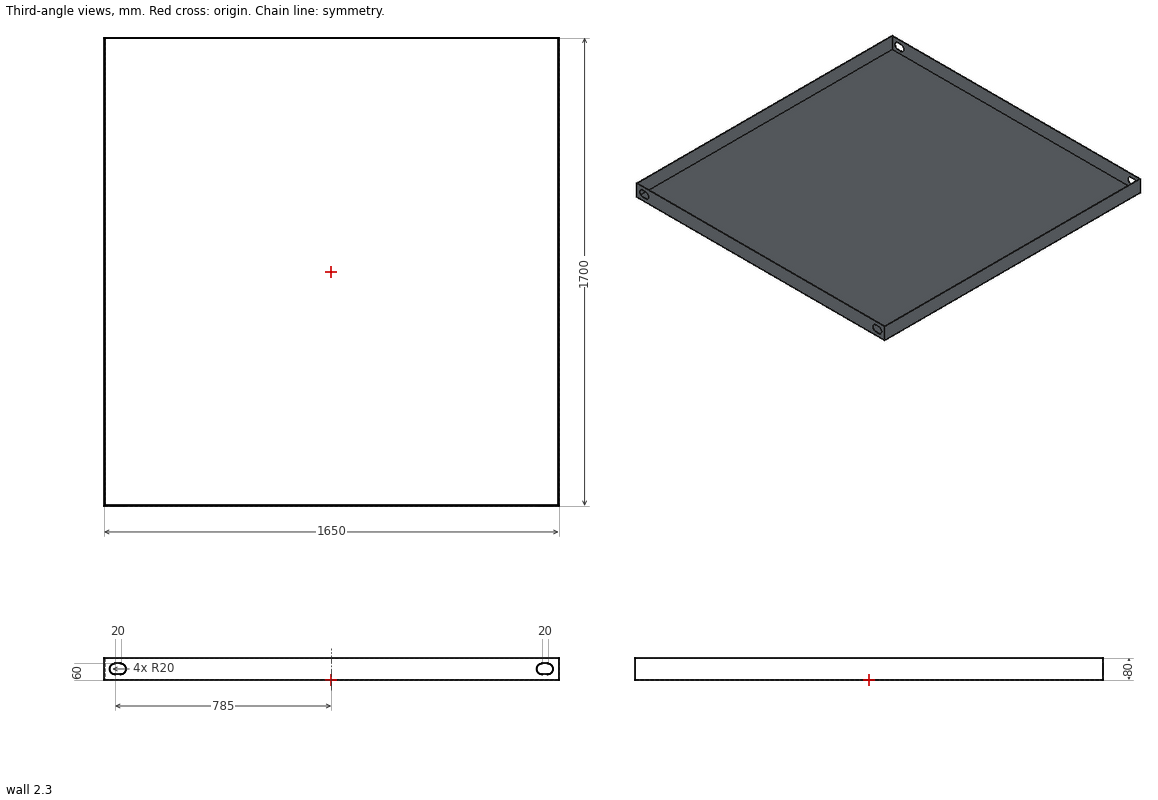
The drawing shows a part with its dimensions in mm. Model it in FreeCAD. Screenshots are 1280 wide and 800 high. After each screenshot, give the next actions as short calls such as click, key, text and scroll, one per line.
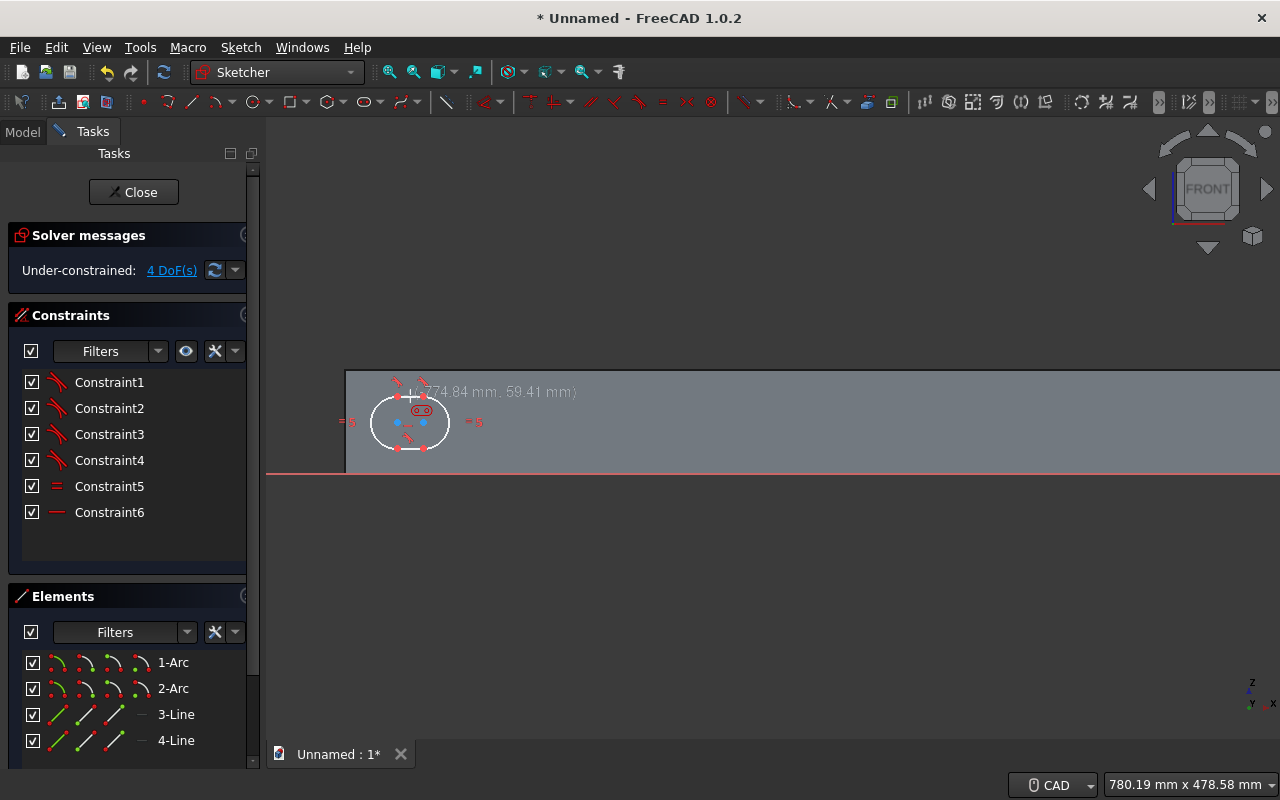
scroll(397, 425, down, 6)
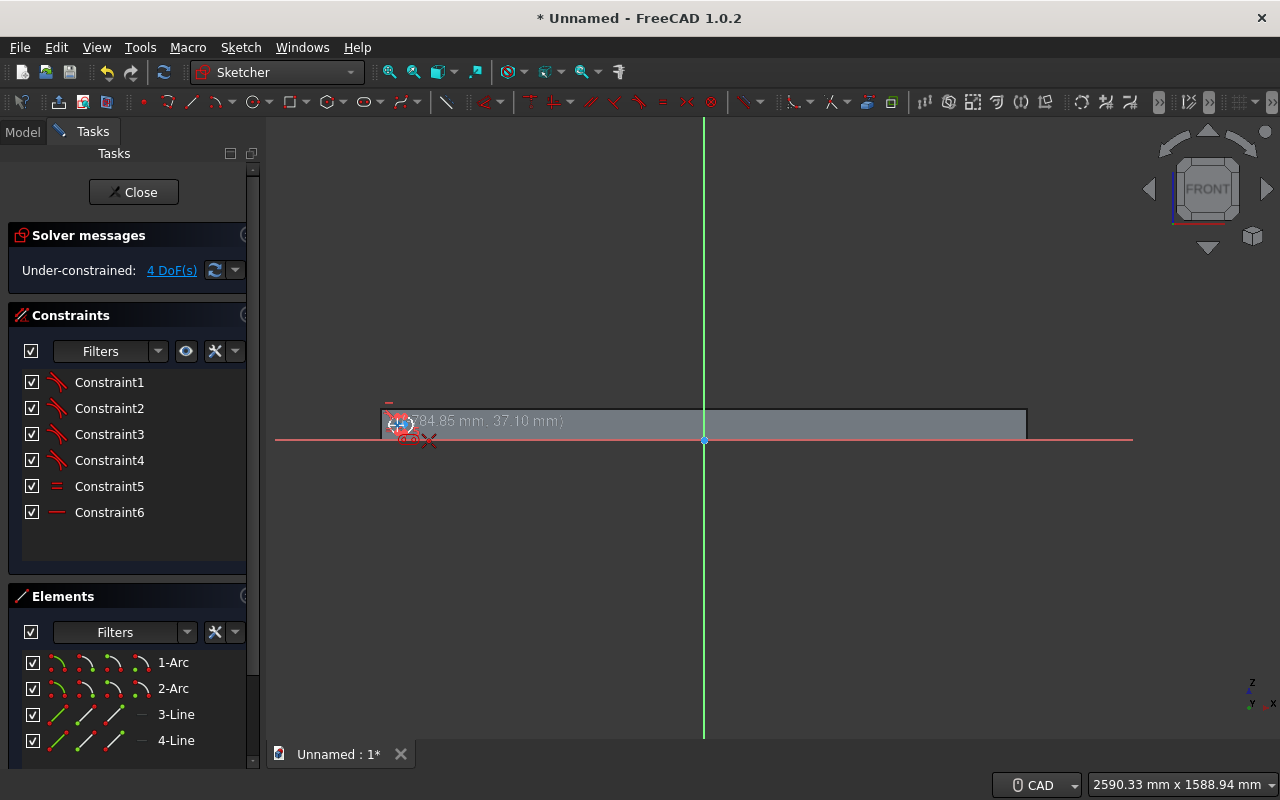
scroll(1004, 425, up, 6)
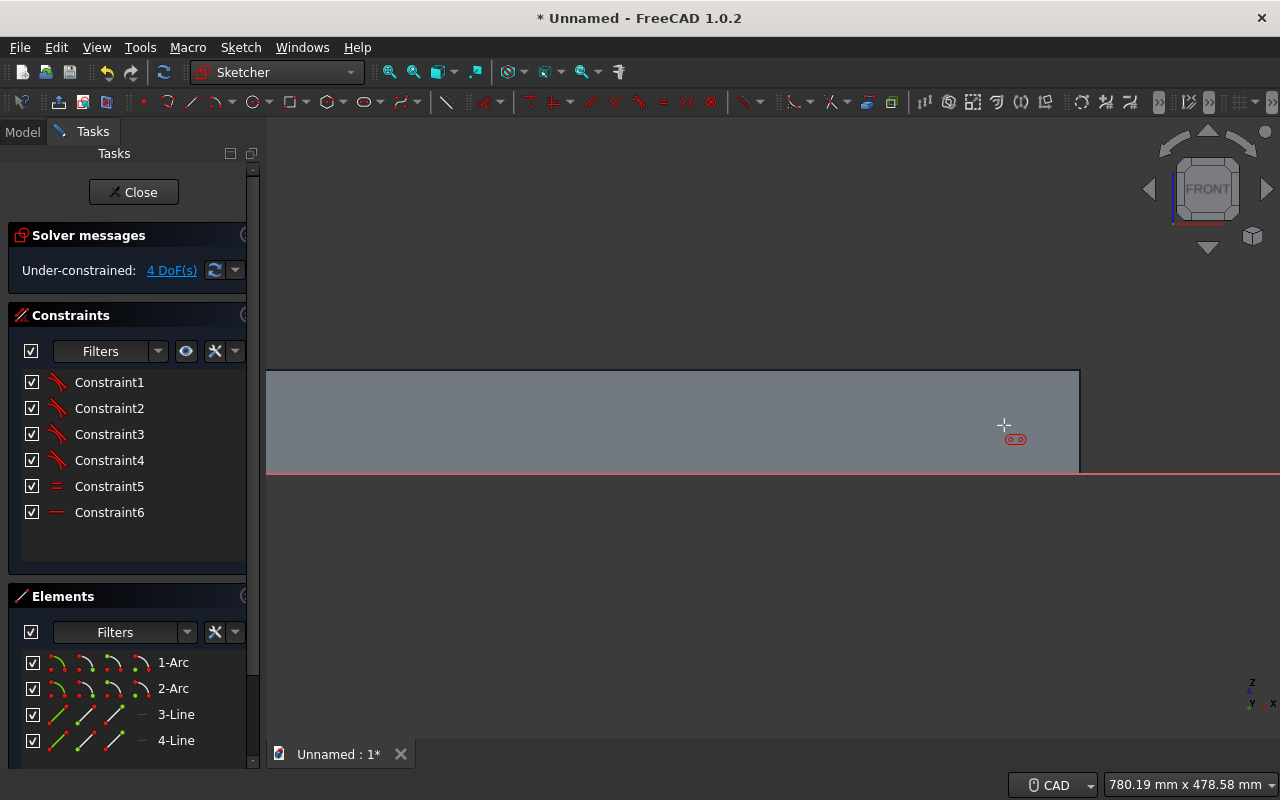
click(1002, 422)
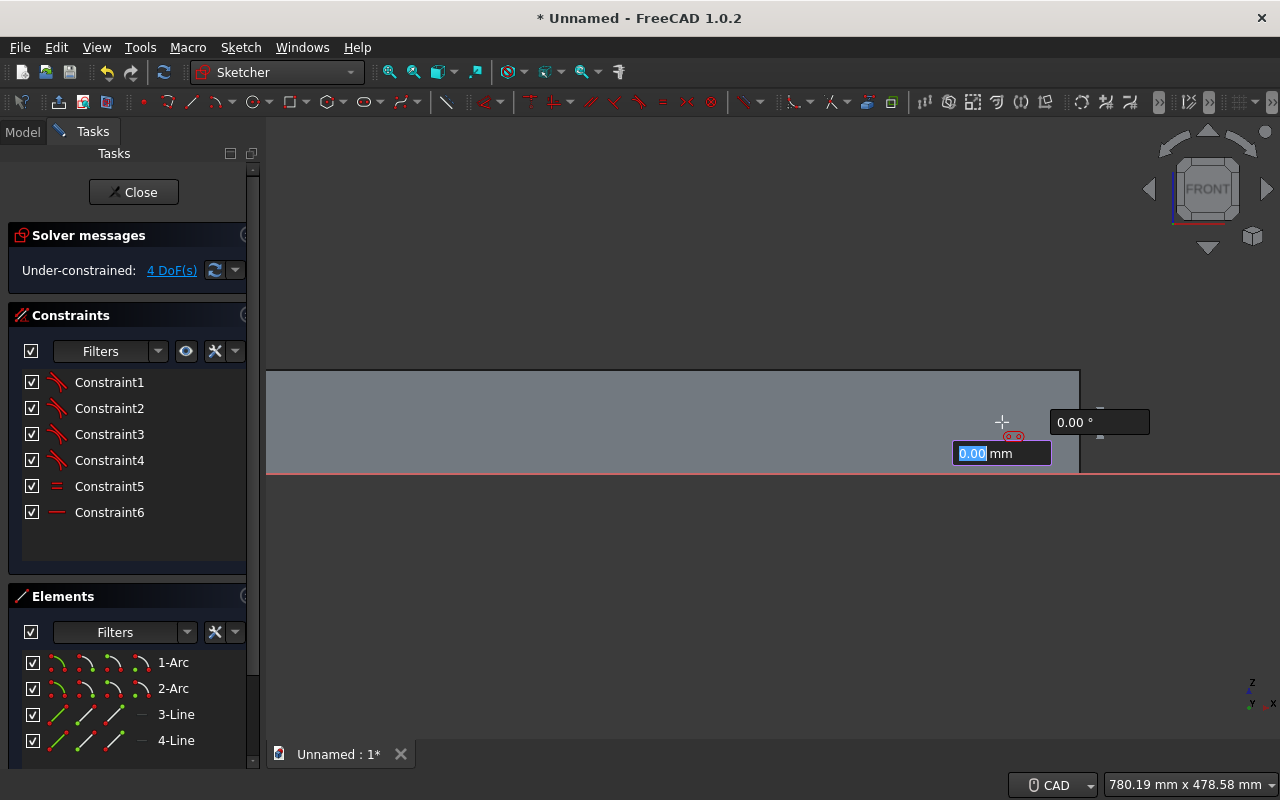
click(1028, 422)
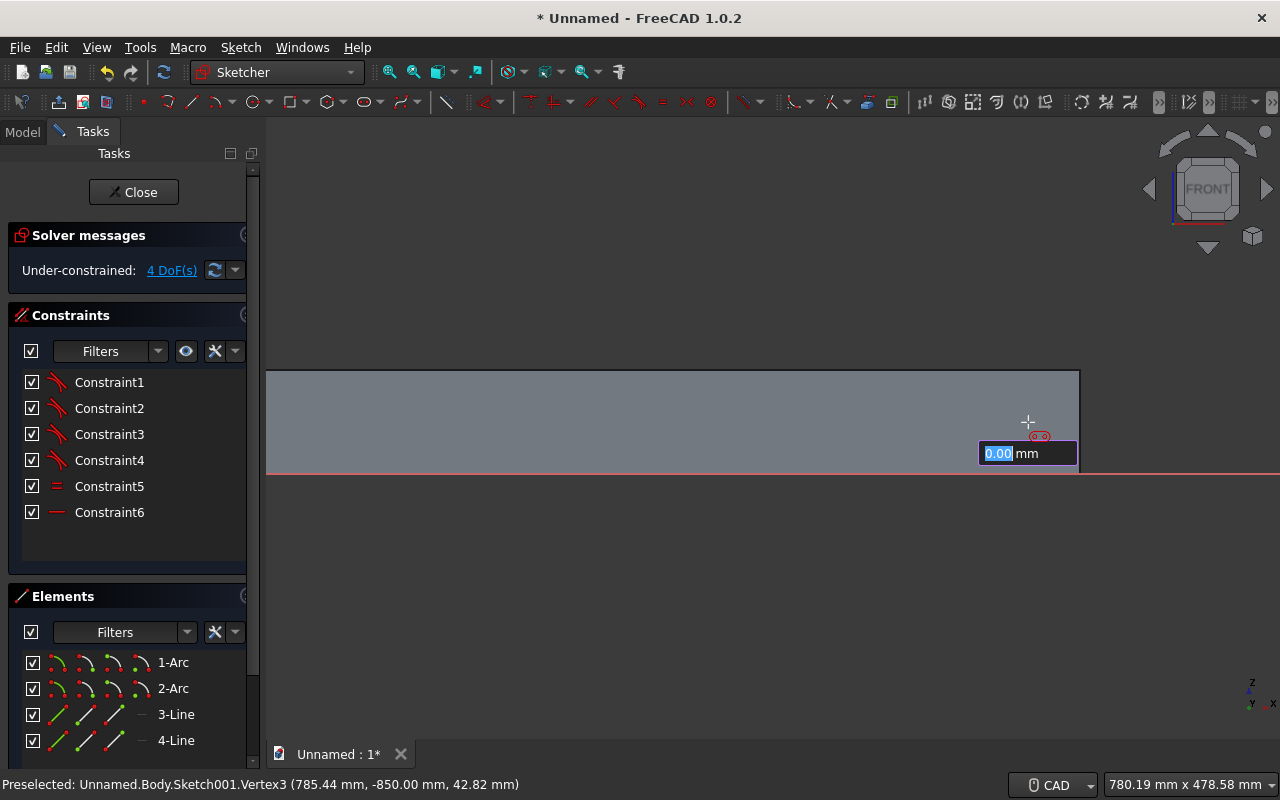
click(1015, 396)
key(Escape)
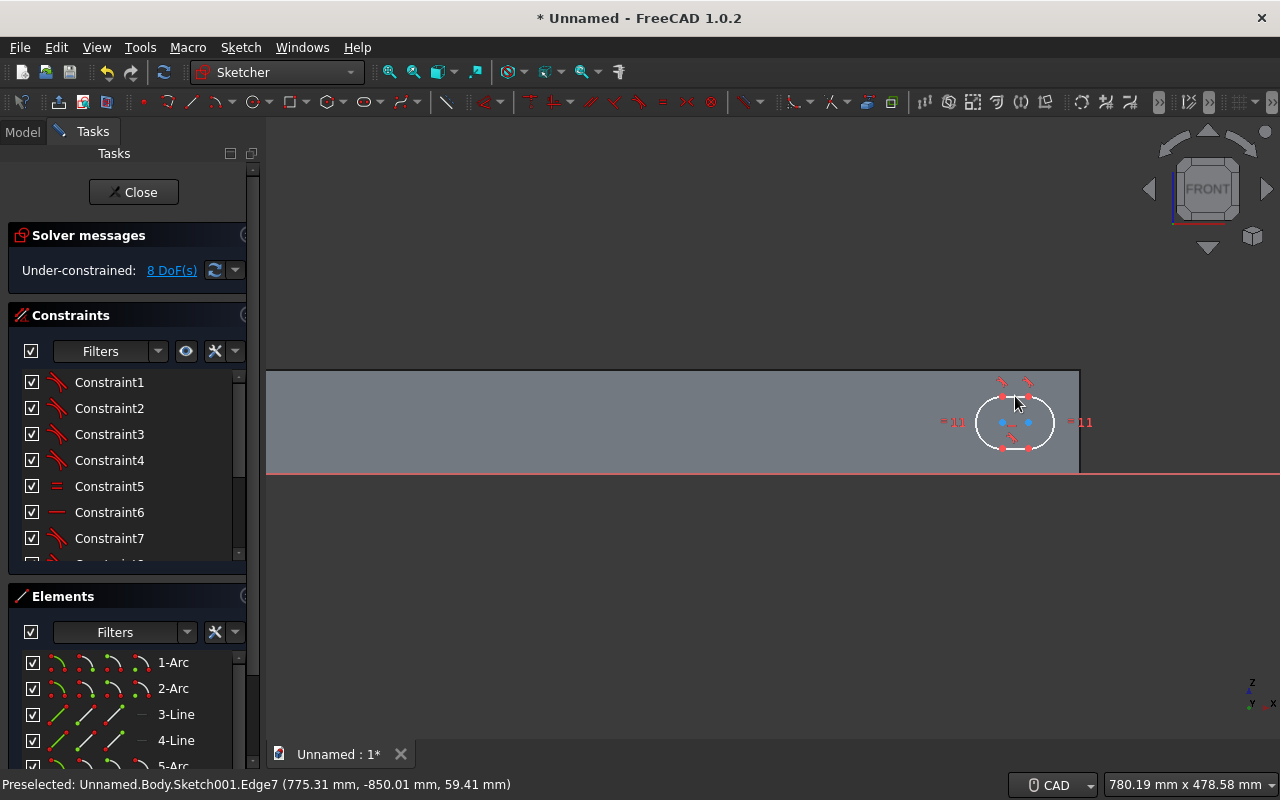
scroll(1005, 425, down, 6)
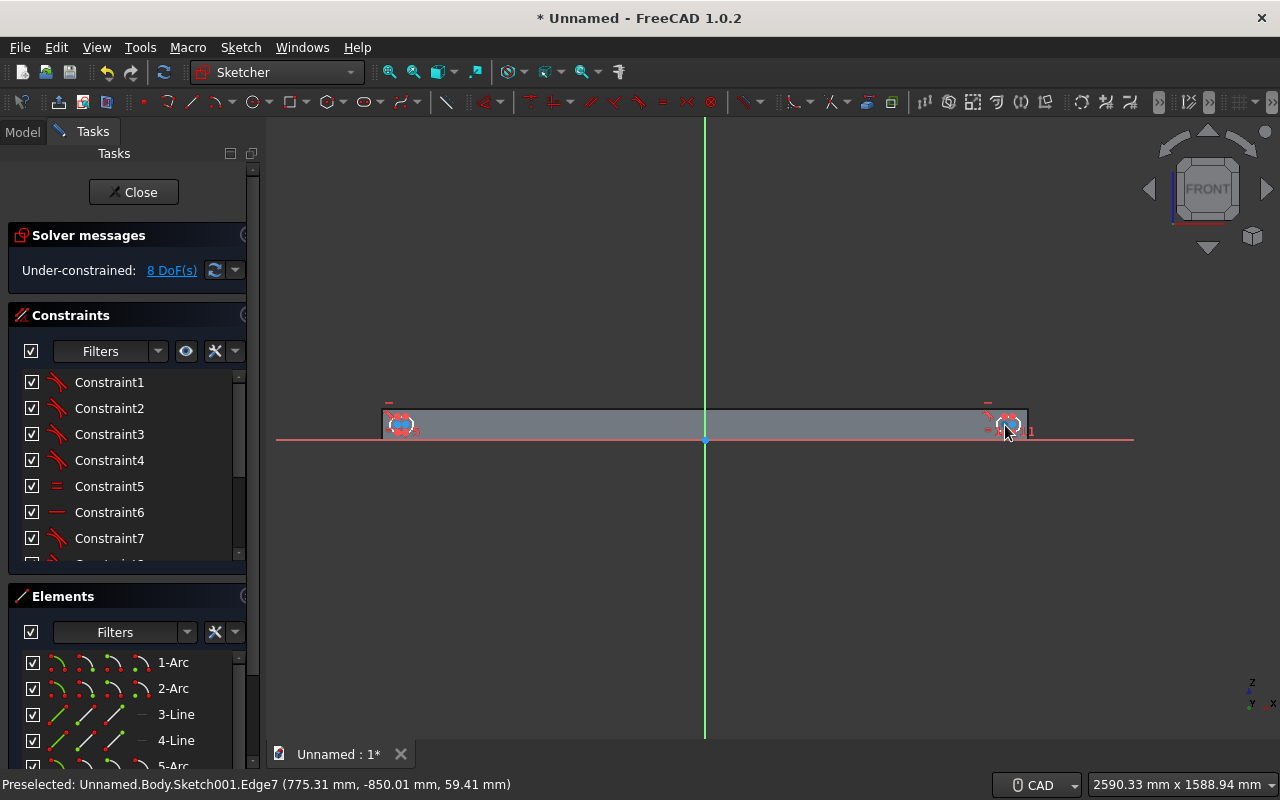
scroll(391, 420, up, 4)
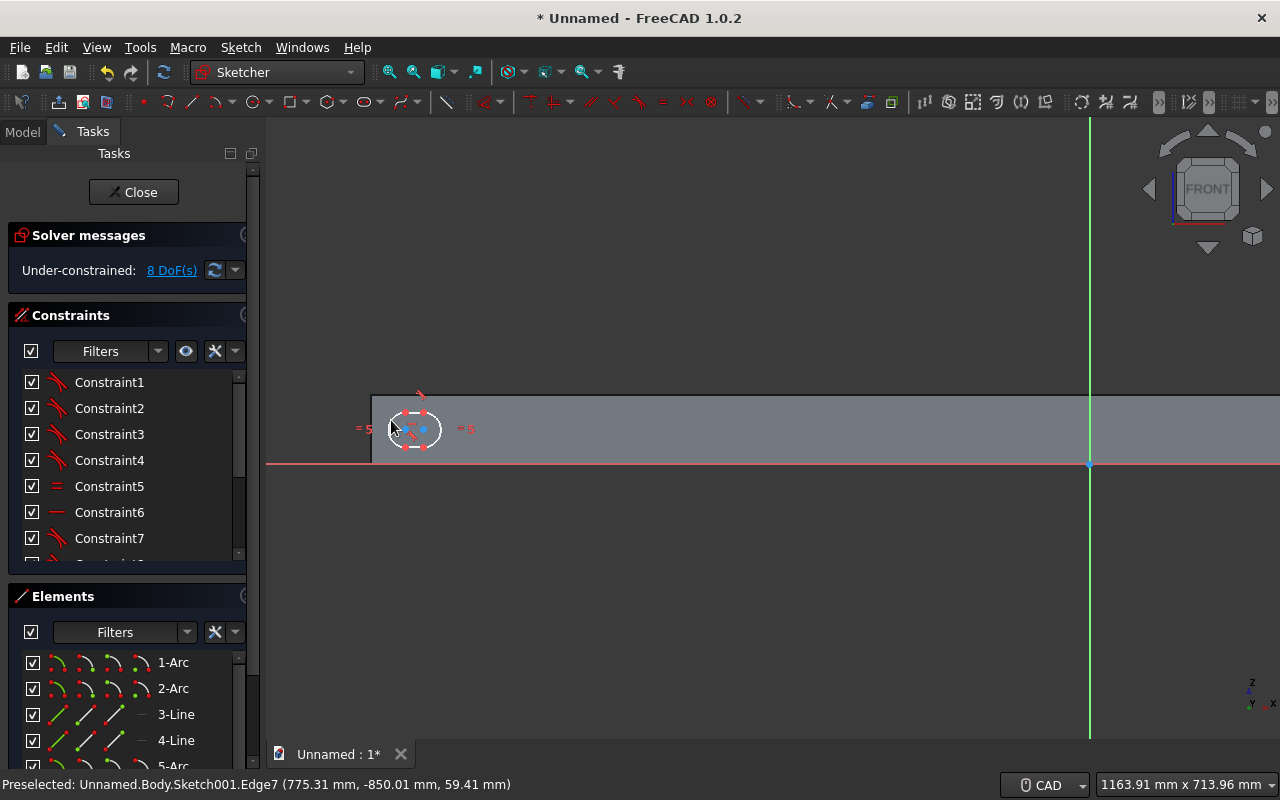
click(392, 420)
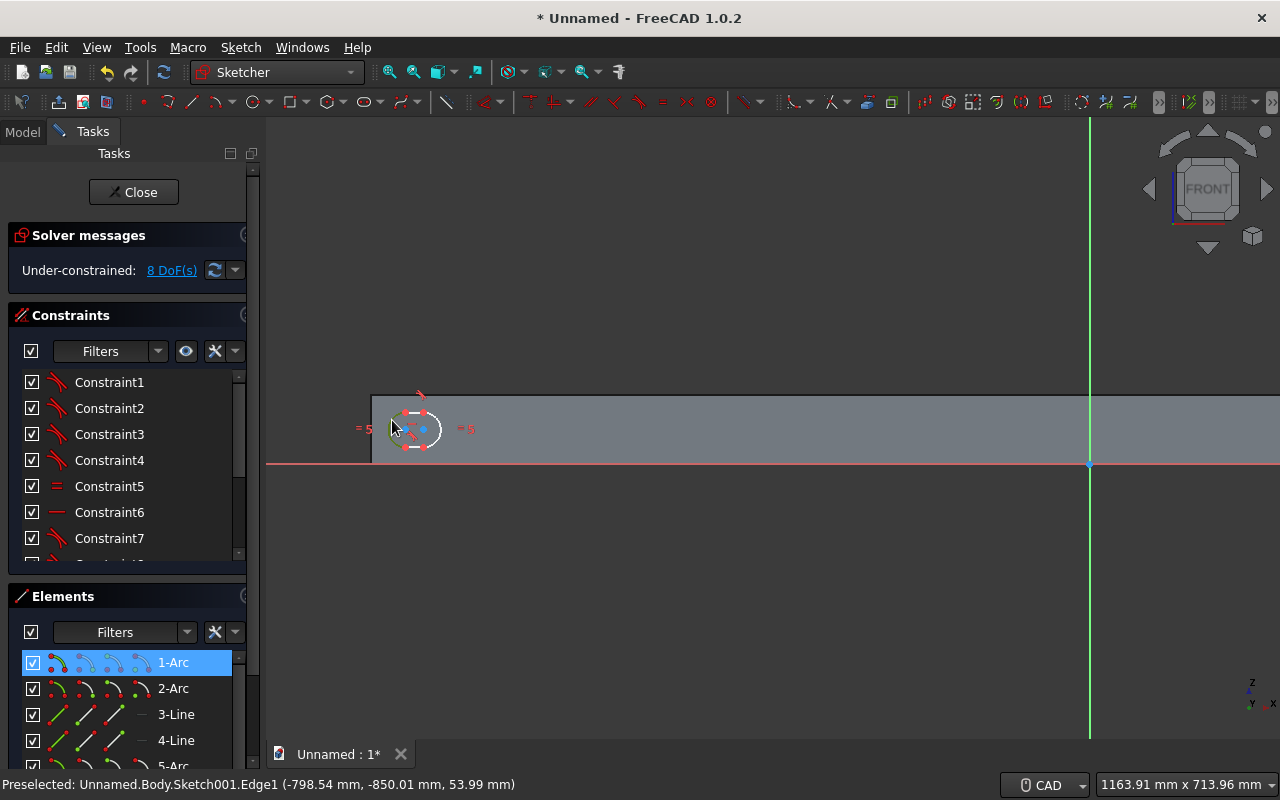
scroll(390, 420, down, 4)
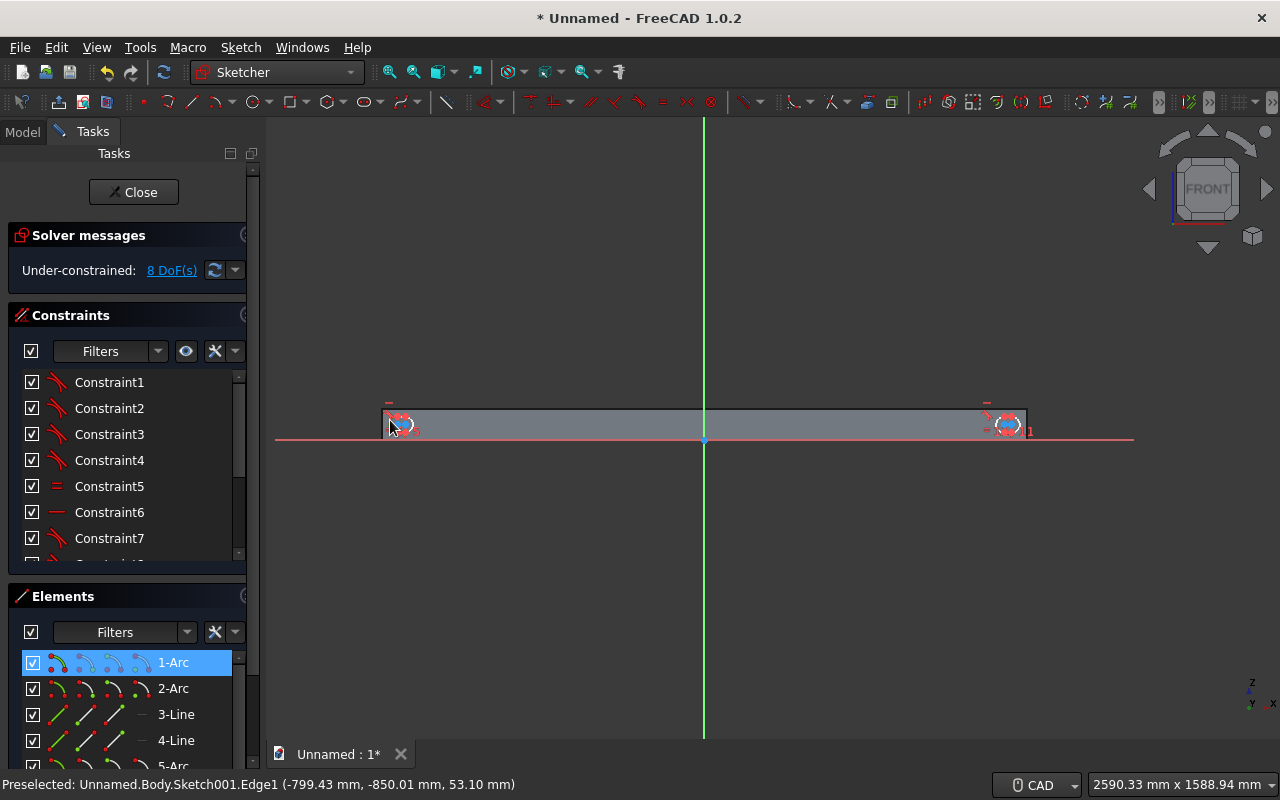
scroll(998, 420, up, 4)